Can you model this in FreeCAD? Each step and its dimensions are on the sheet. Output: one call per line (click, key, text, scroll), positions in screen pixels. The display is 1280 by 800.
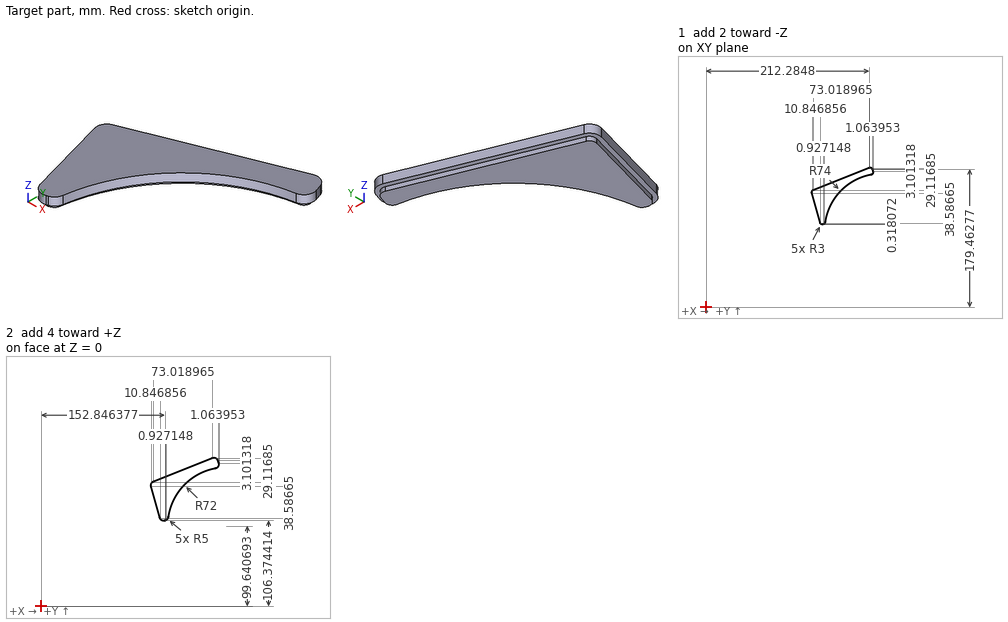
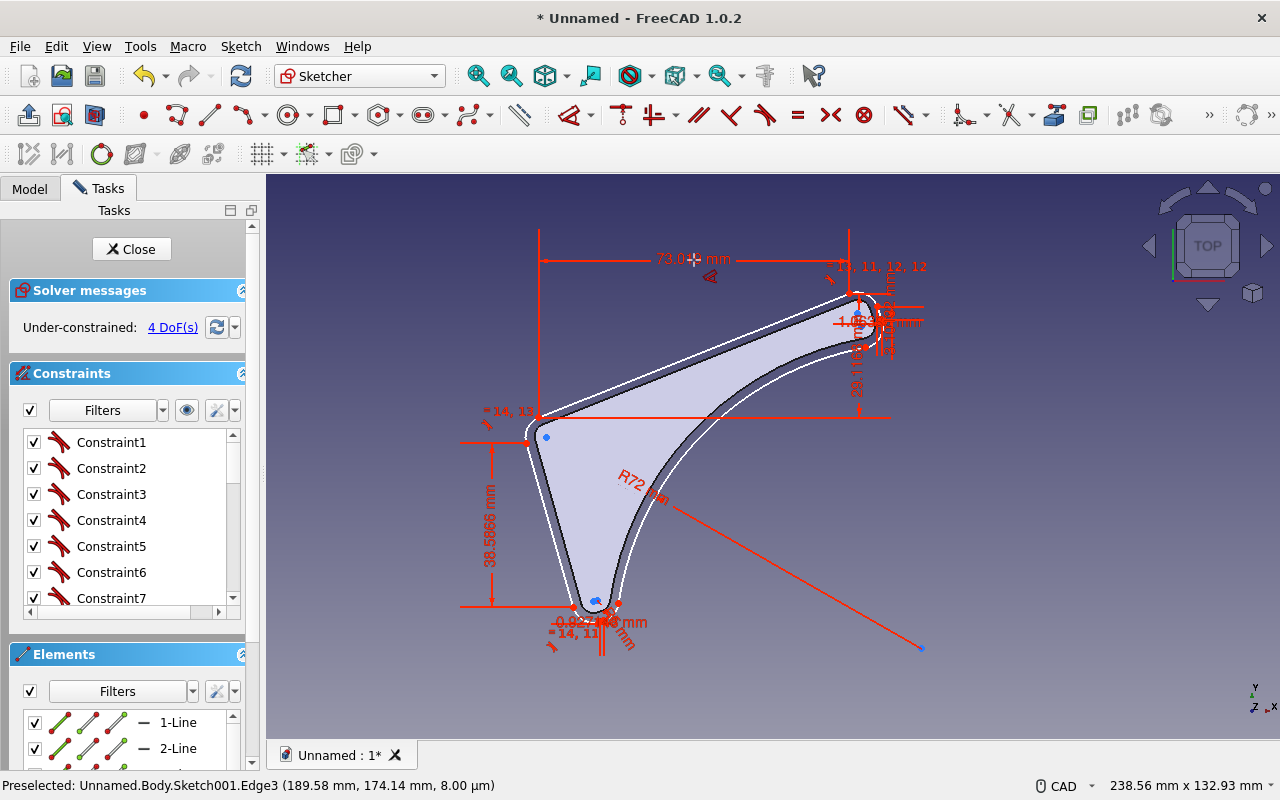
click(540, 492)
click(550, 665)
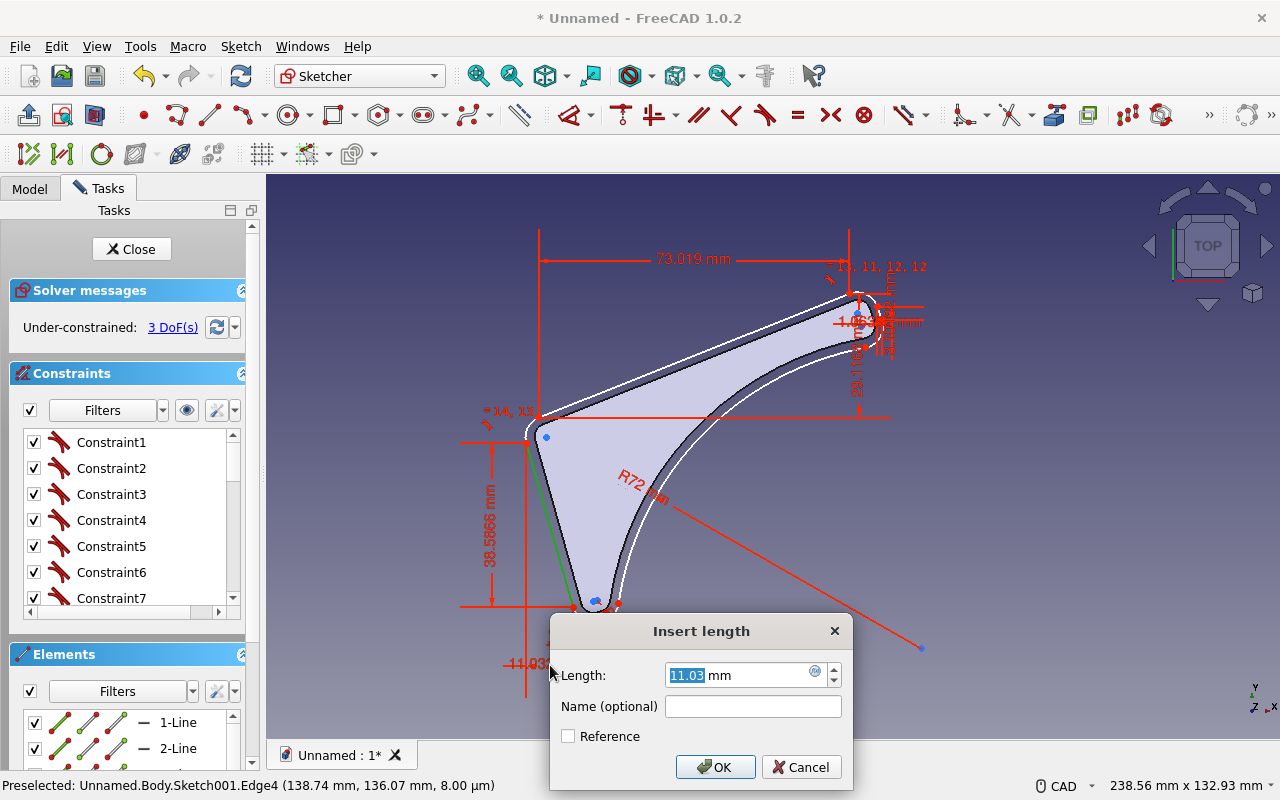
text(10.846856)
key(Return)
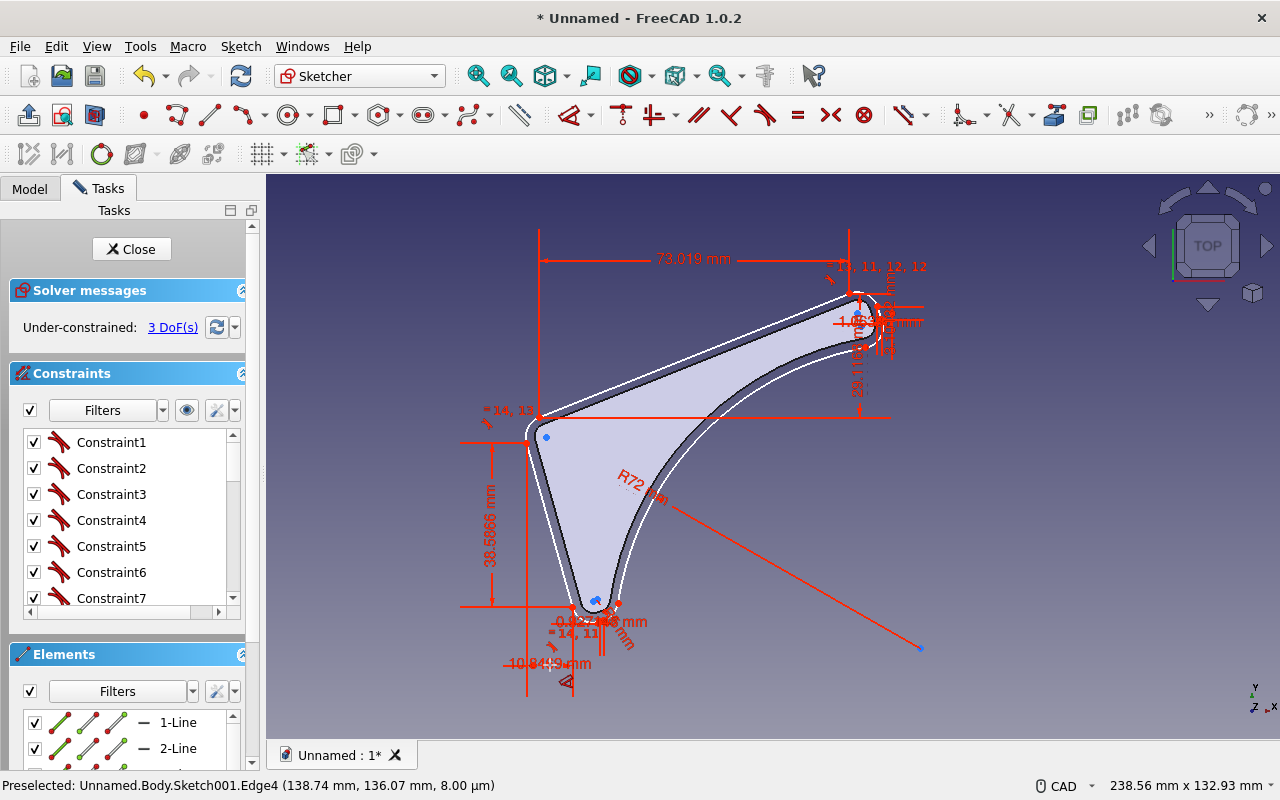
click(921, 649)
click(955, 680)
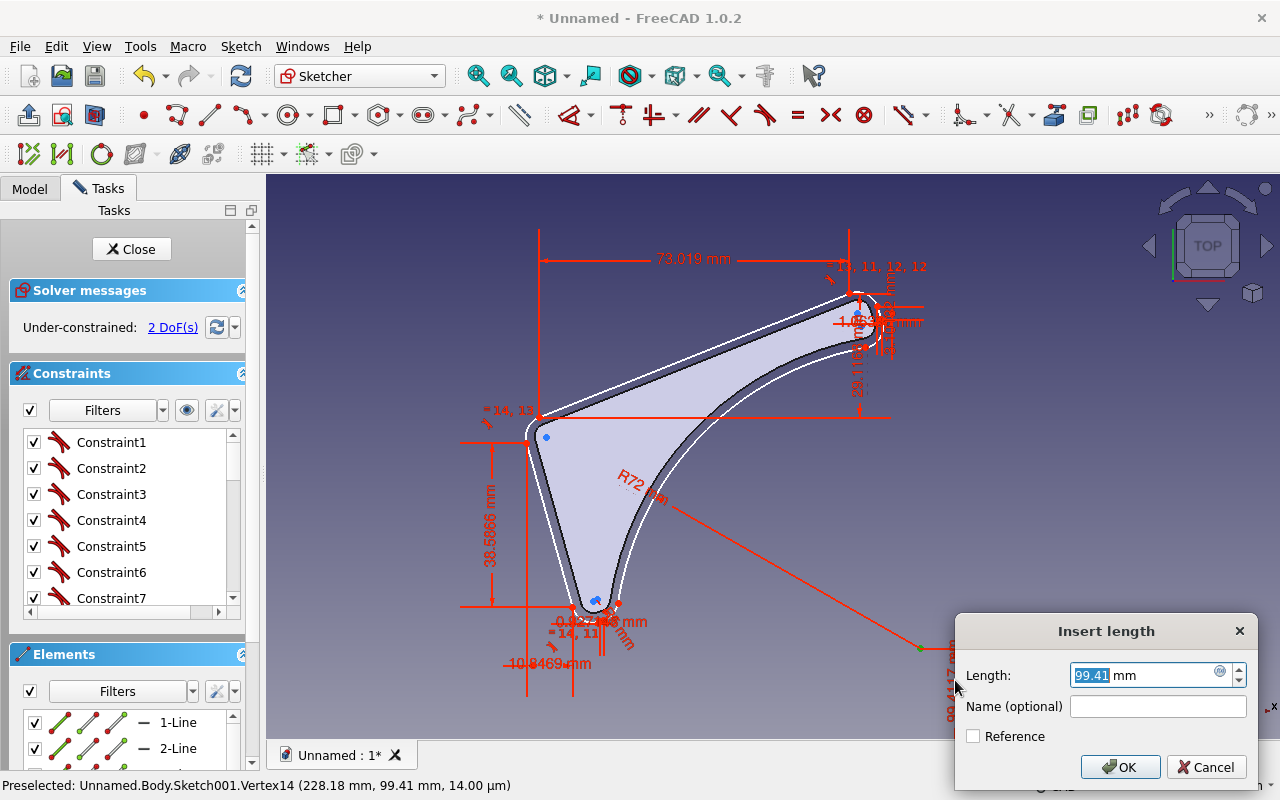
text(99.640693)
key(Return)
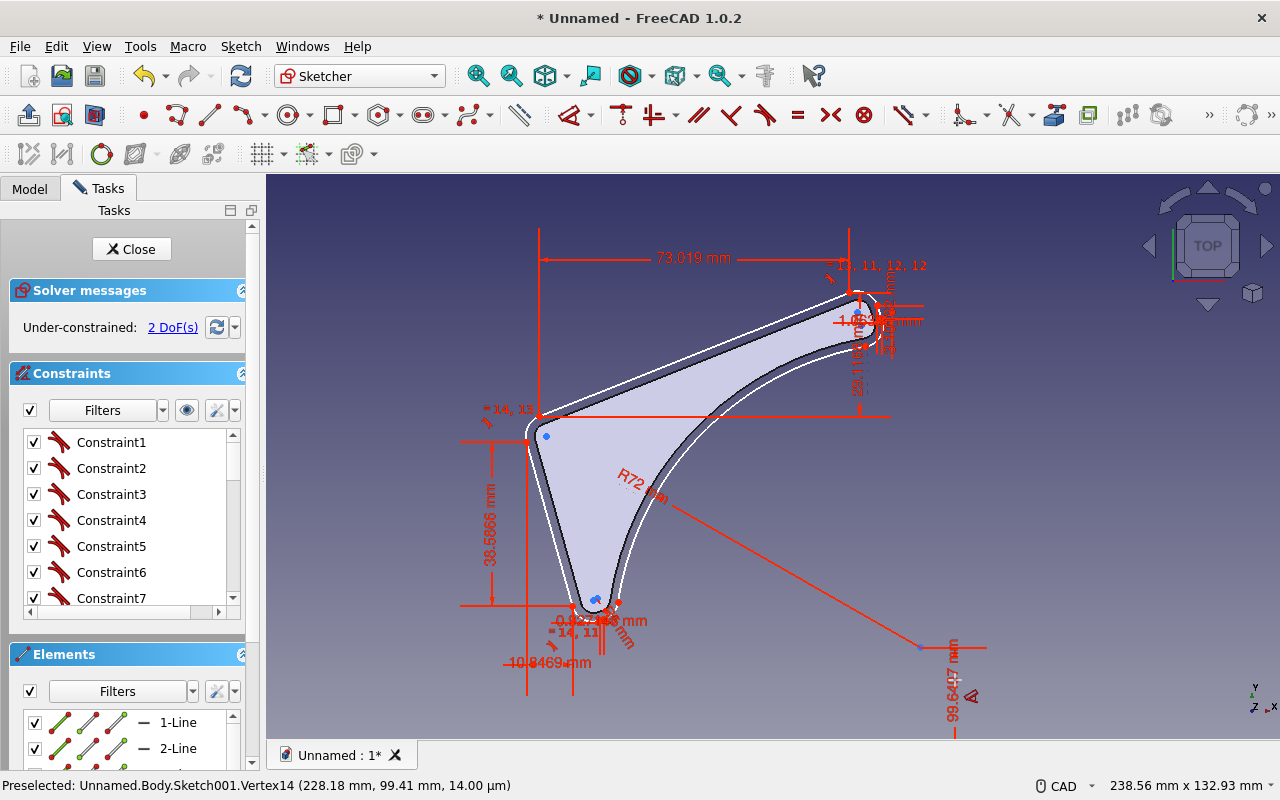
scroll(600, 620, up, 6)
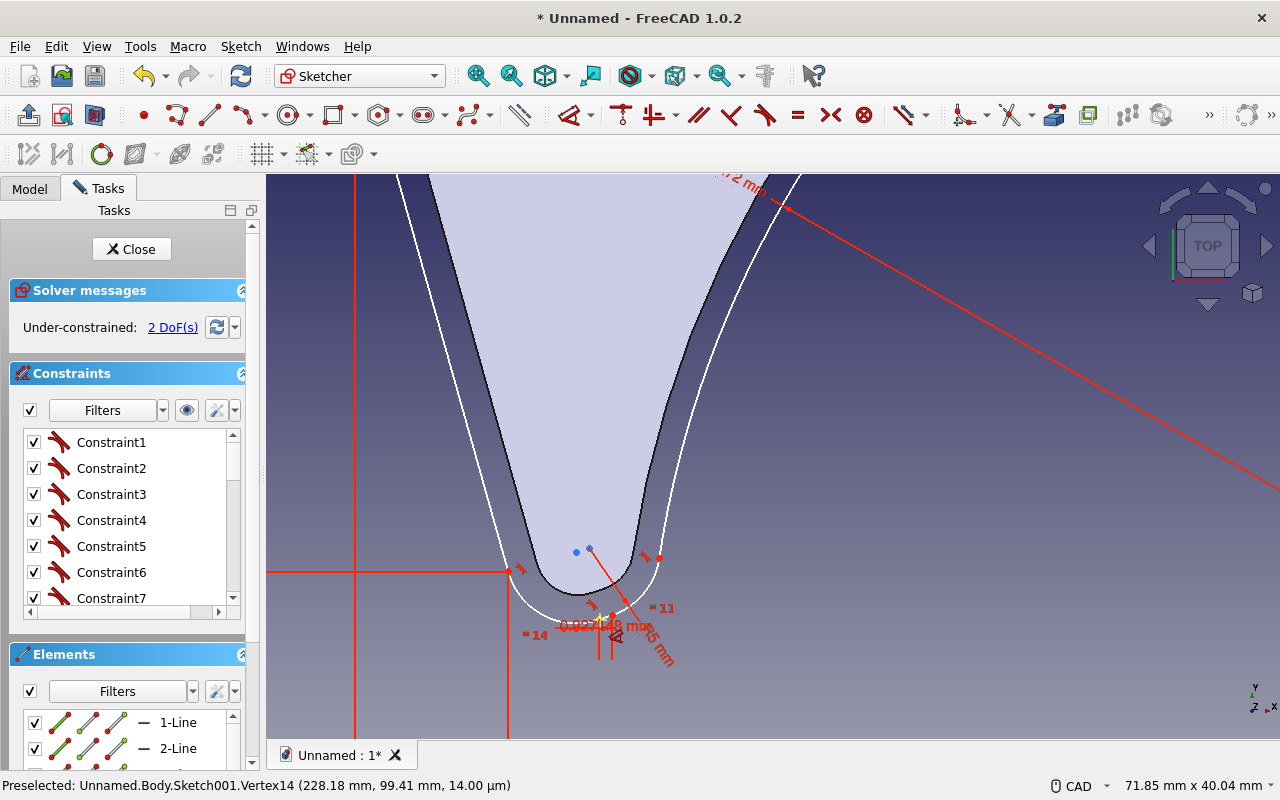
click(599, 620)
click(447, 586)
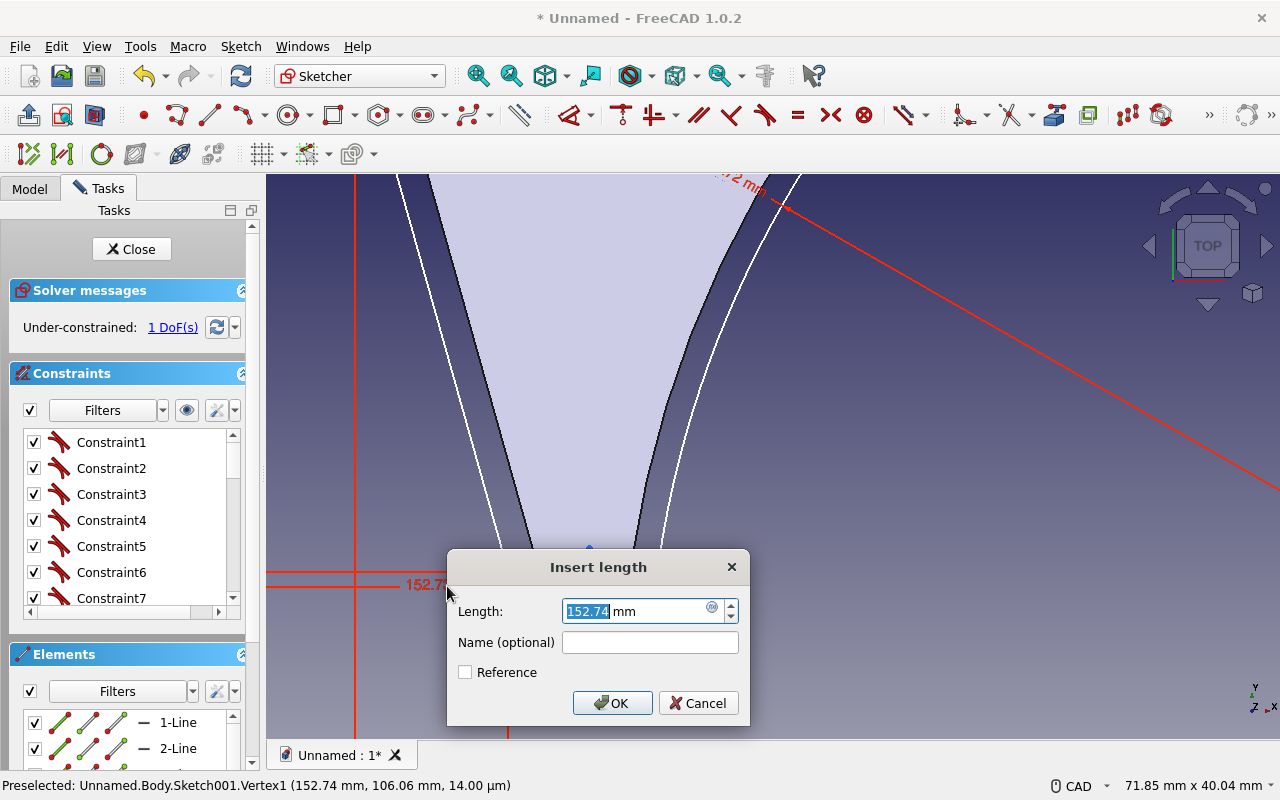
text(152.846377)
key(Return)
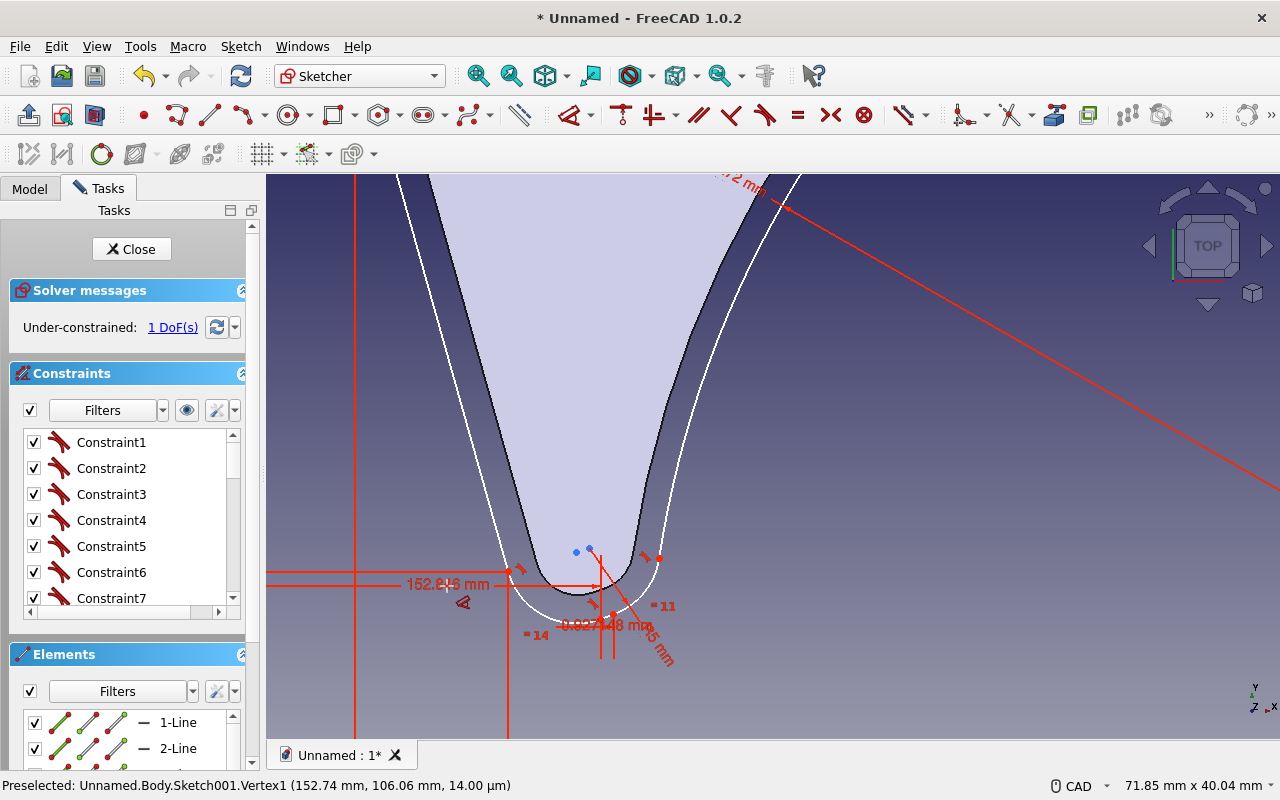
click(614, 614)
click(648, 685)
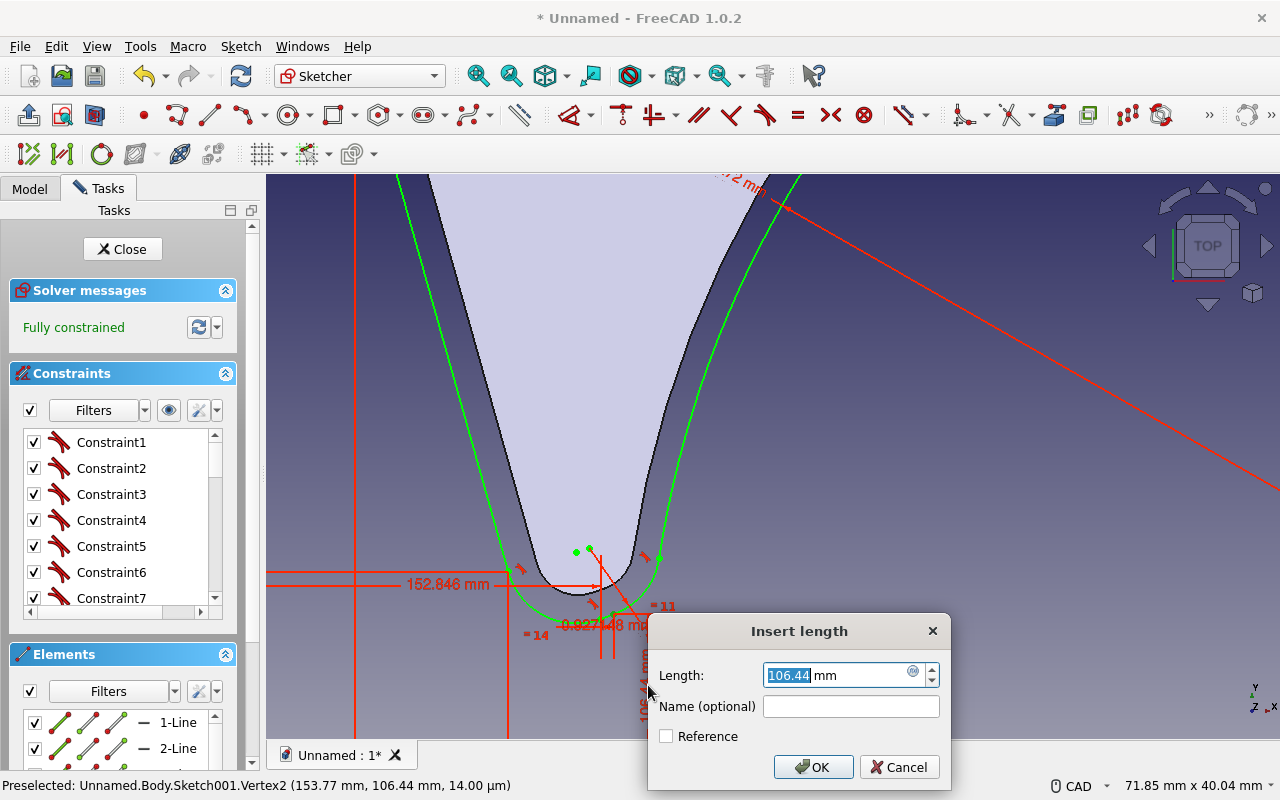
text(106.374414)
key(Return)
key(Escape)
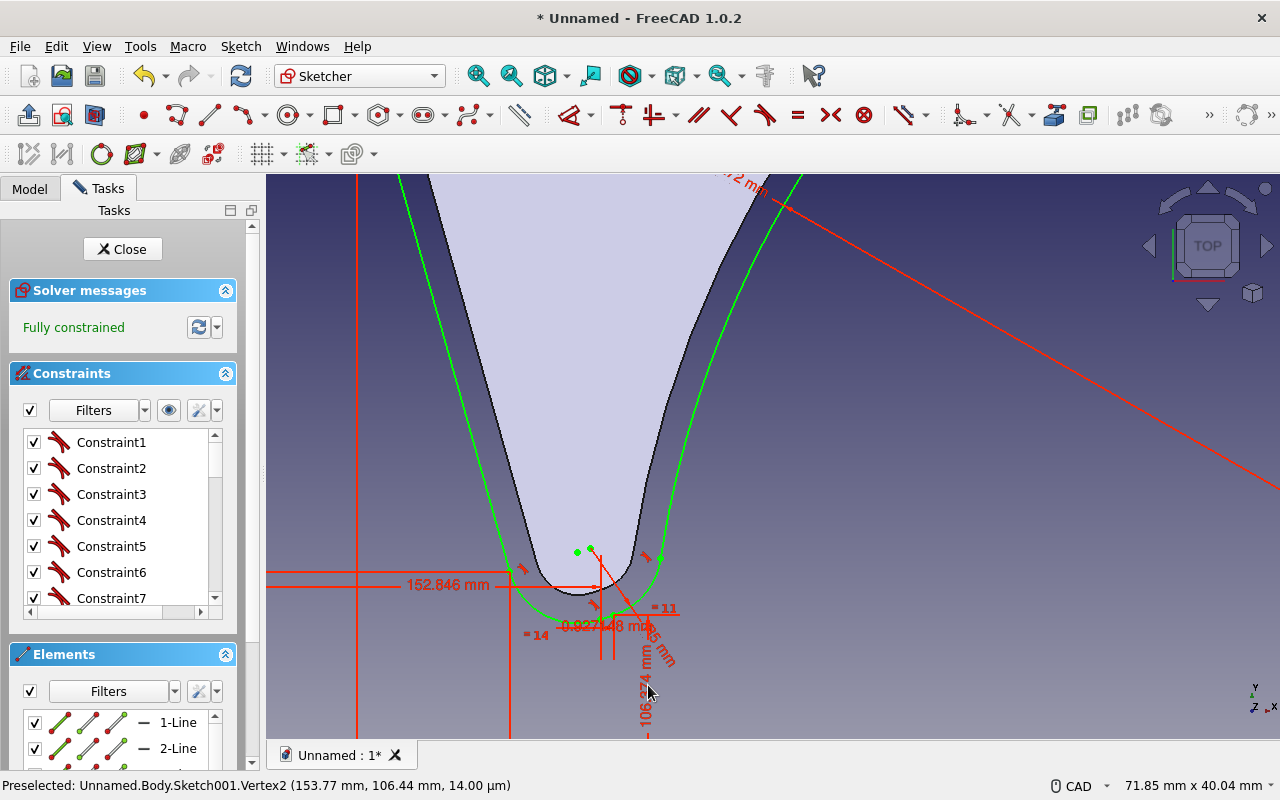
click(123, 249)